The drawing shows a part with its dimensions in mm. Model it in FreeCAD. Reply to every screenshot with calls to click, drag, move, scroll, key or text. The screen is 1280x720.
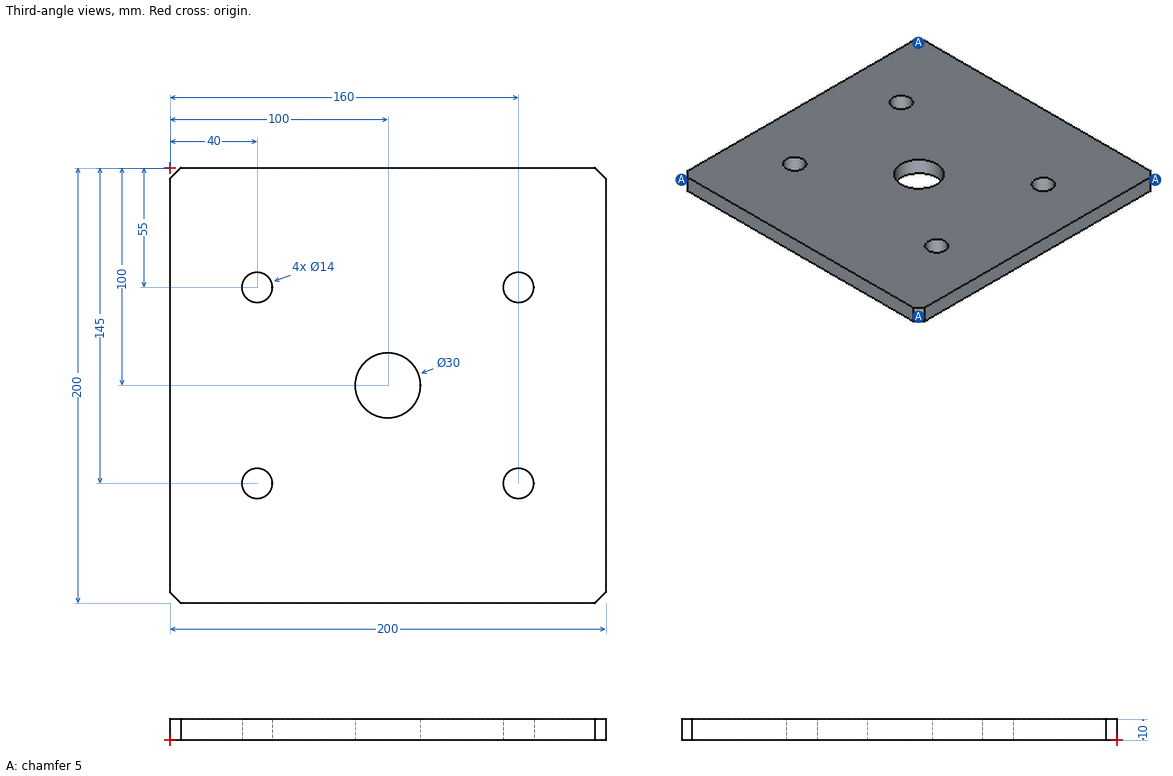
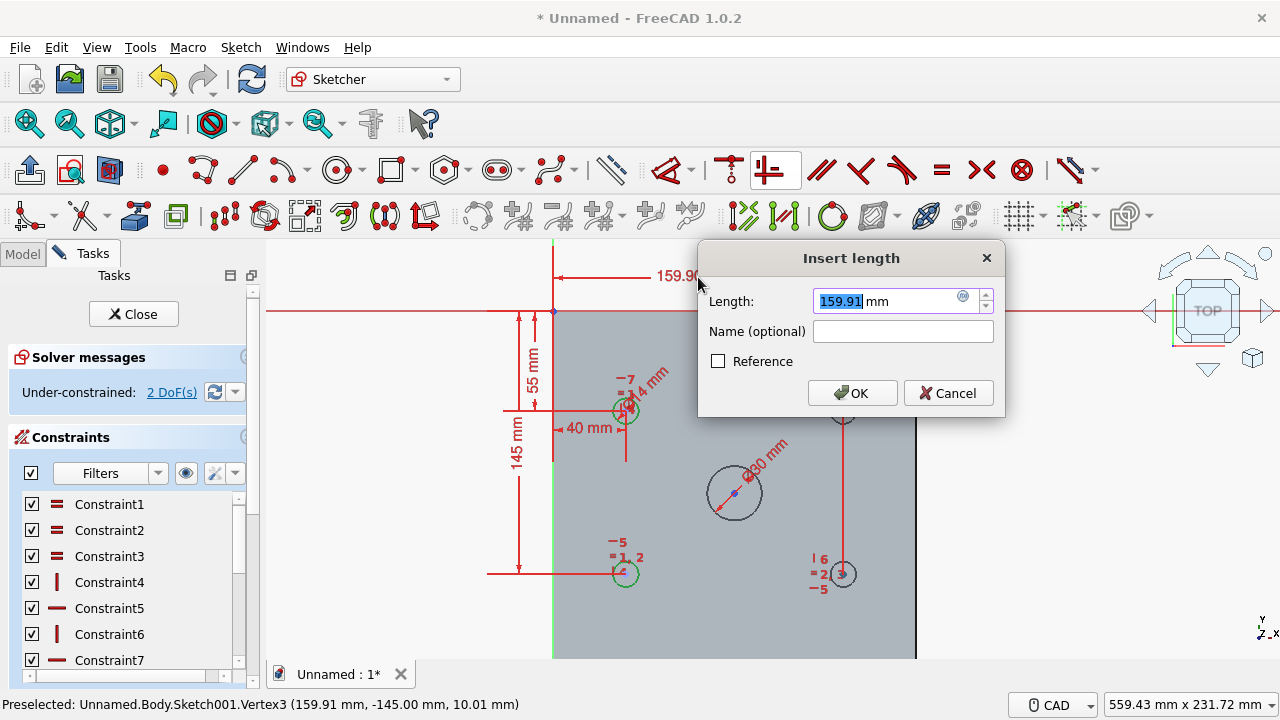
text(160)
key(Return)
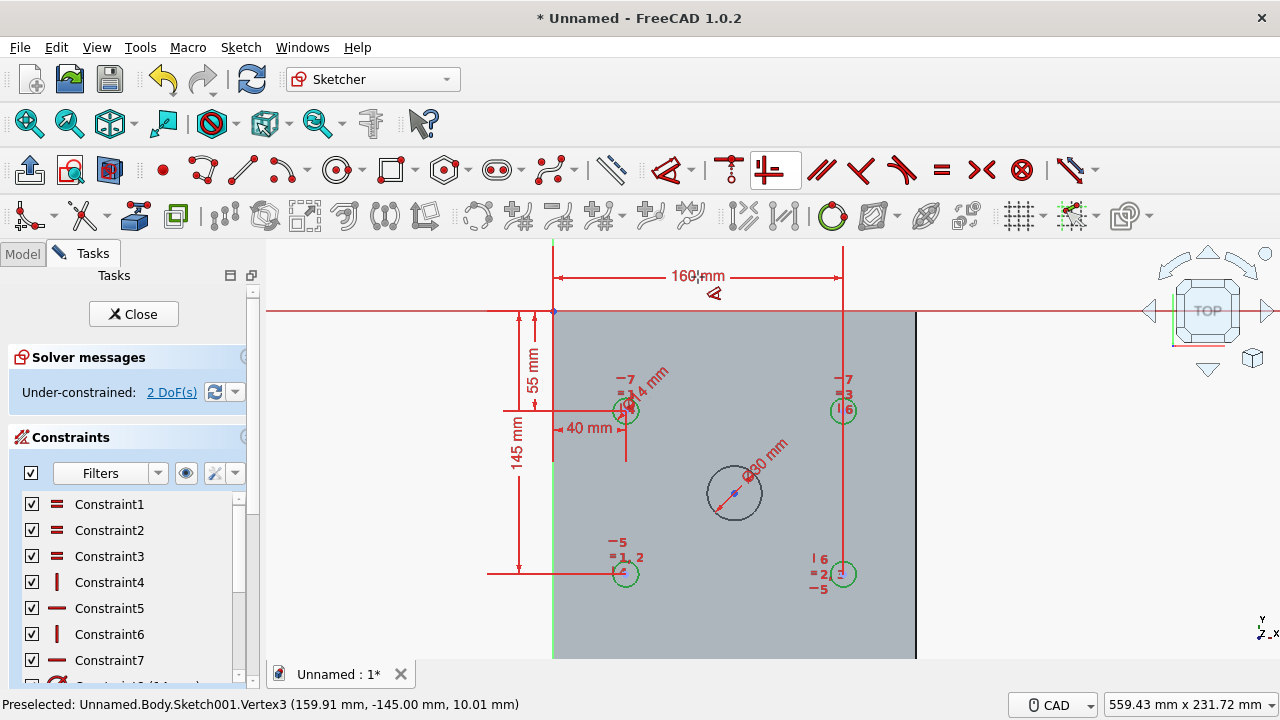
click(735, 493)
click(602, 277)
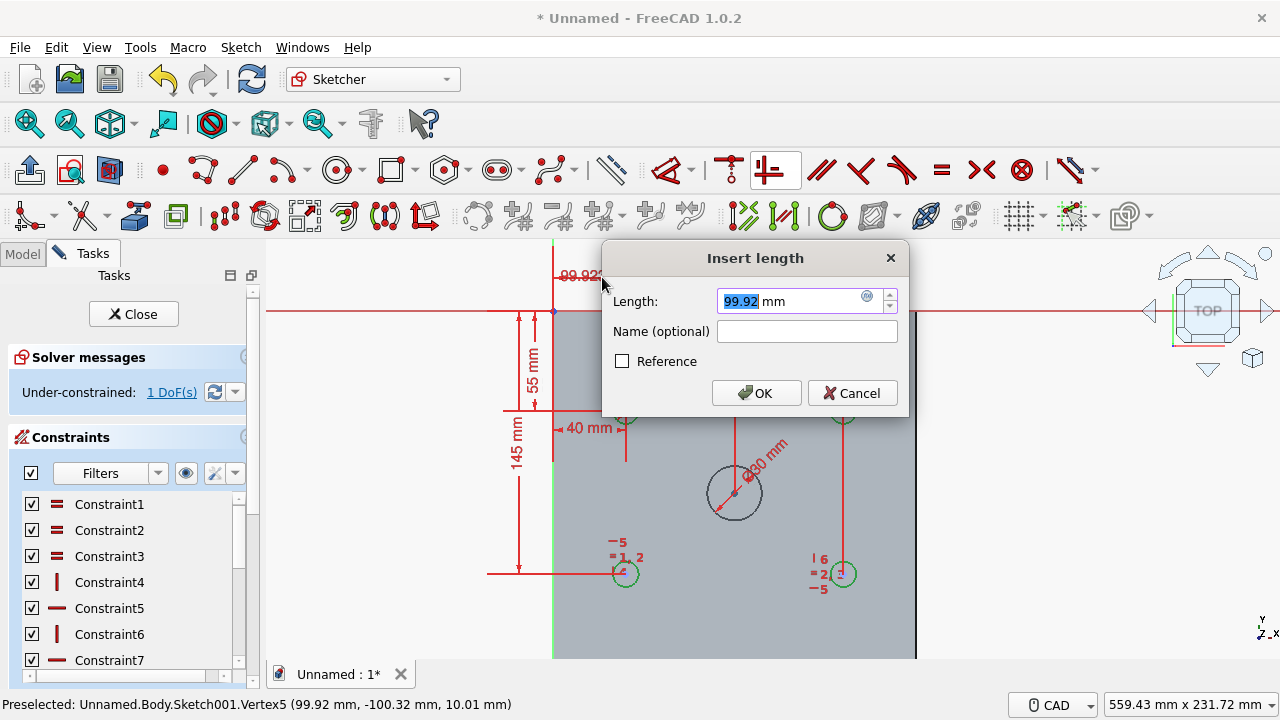
text(100)
key(Return)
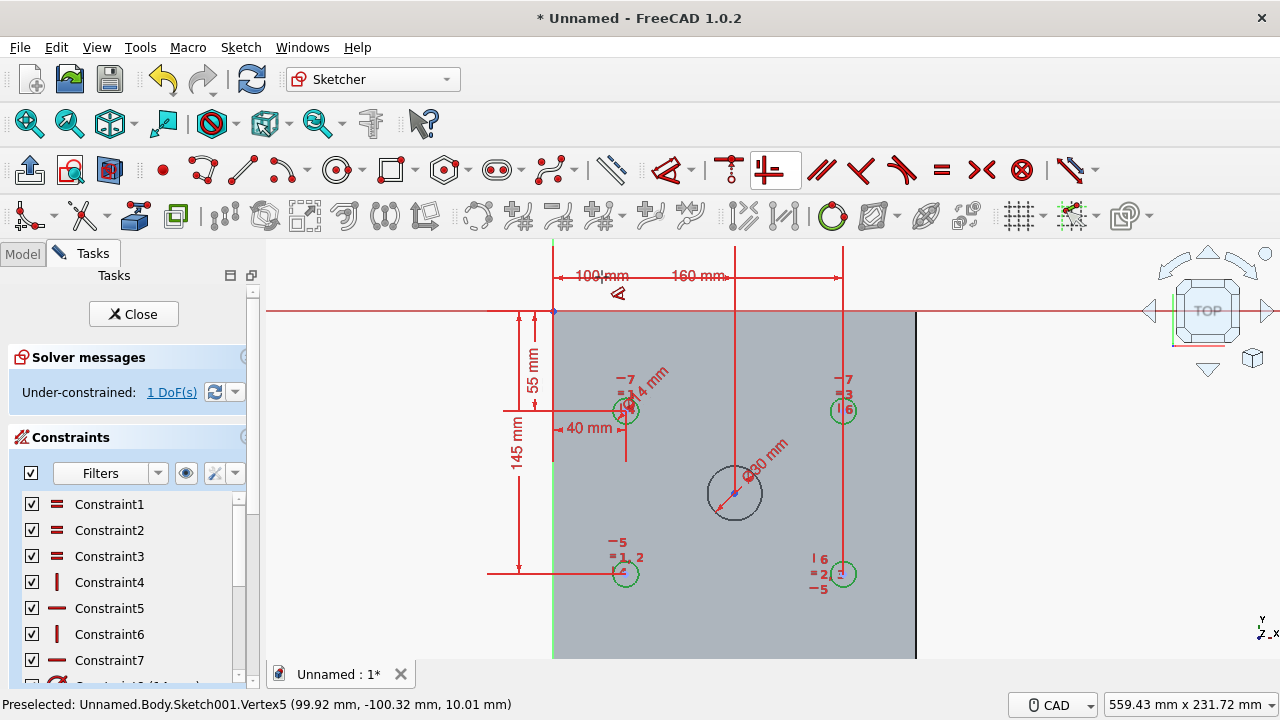
click(735, 493)
click(519, 402)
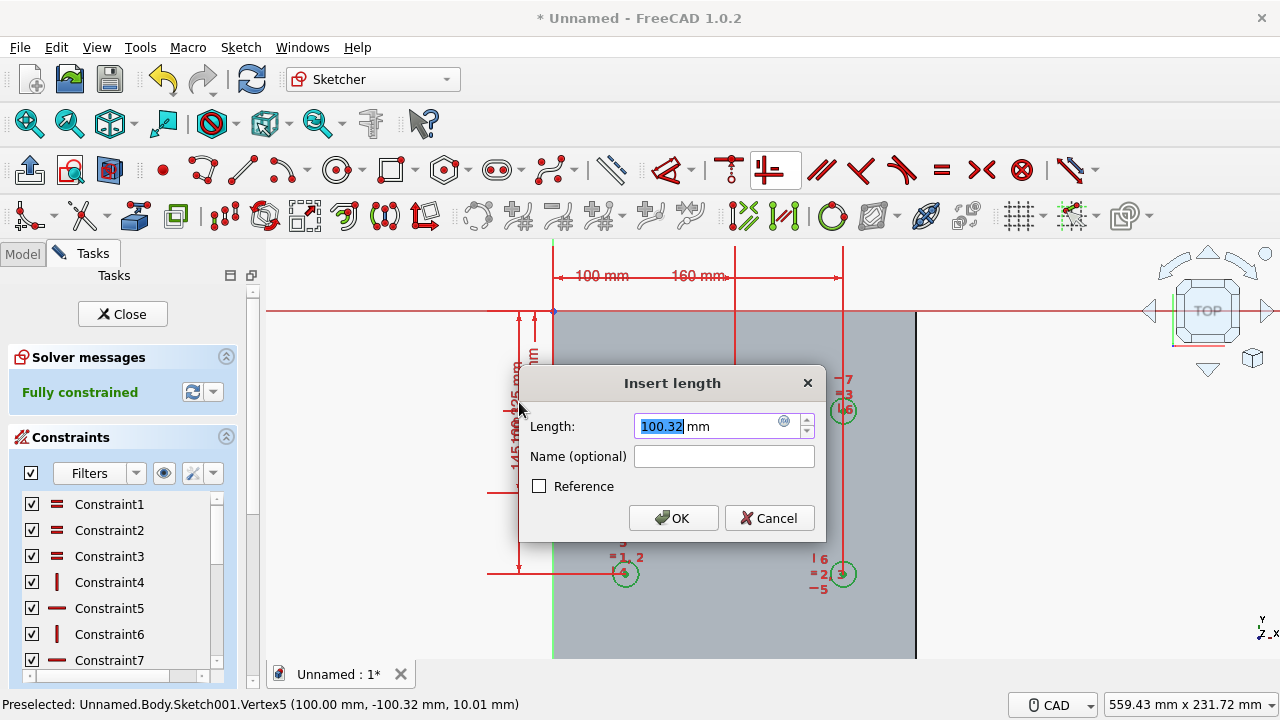
text(100)
key(Return)
key(Escape)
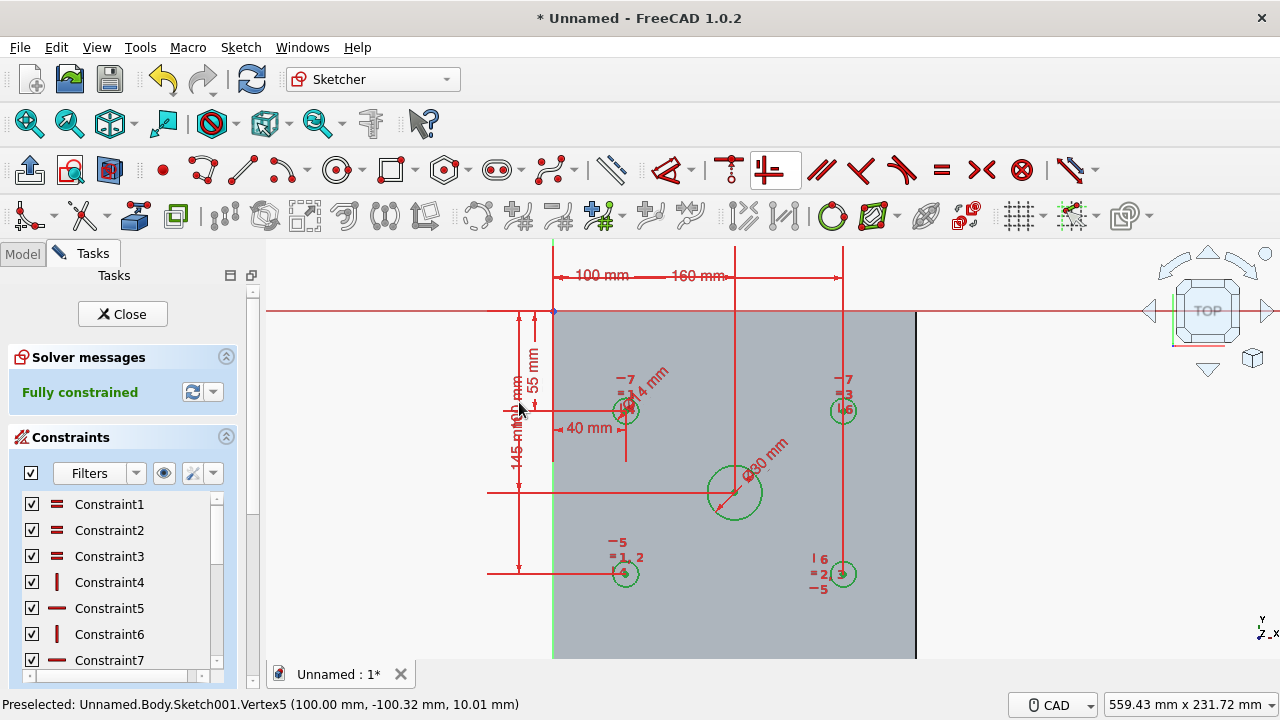
click(123, 314)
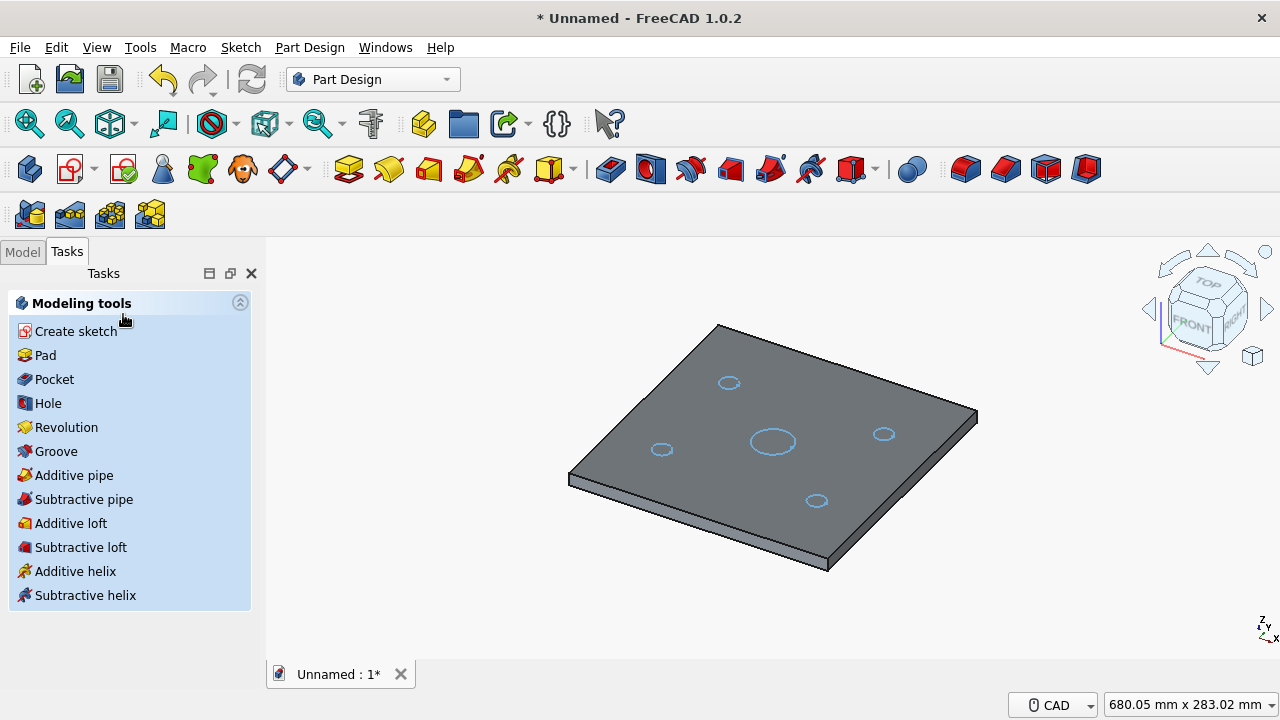
click(612, 170)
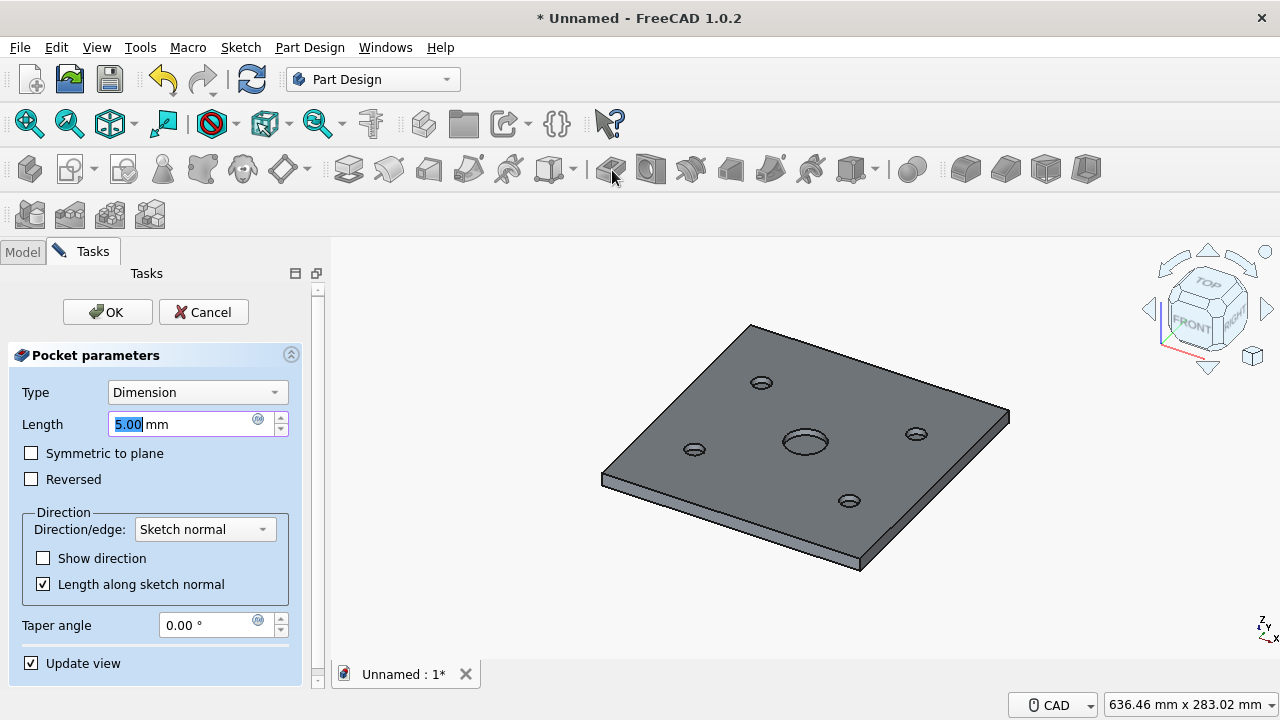
click(198, 392)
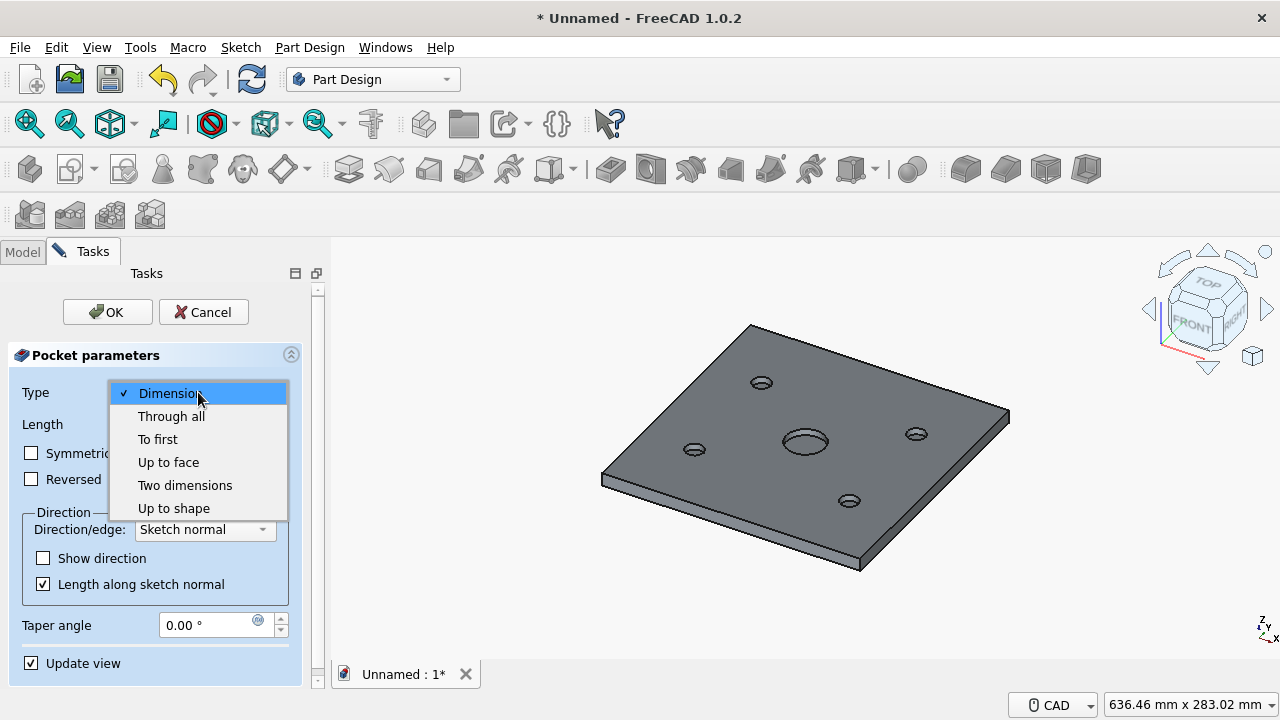
click(198, 416)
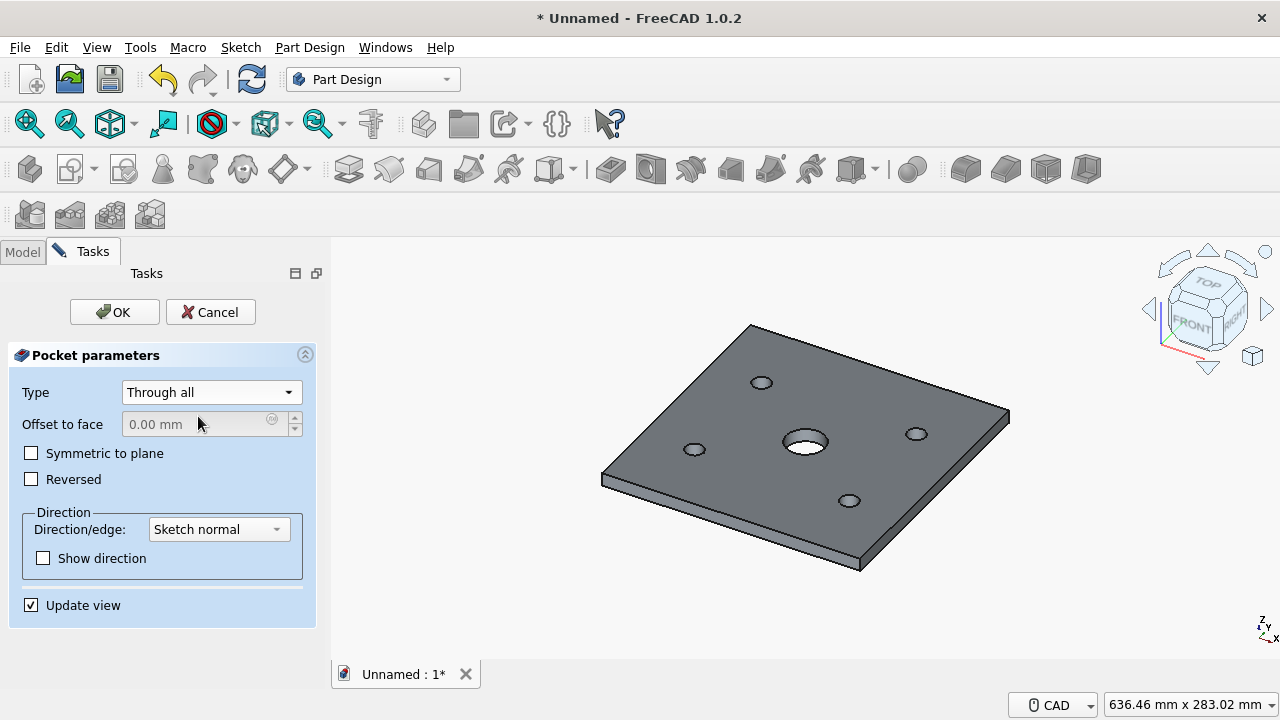
click(115, 312)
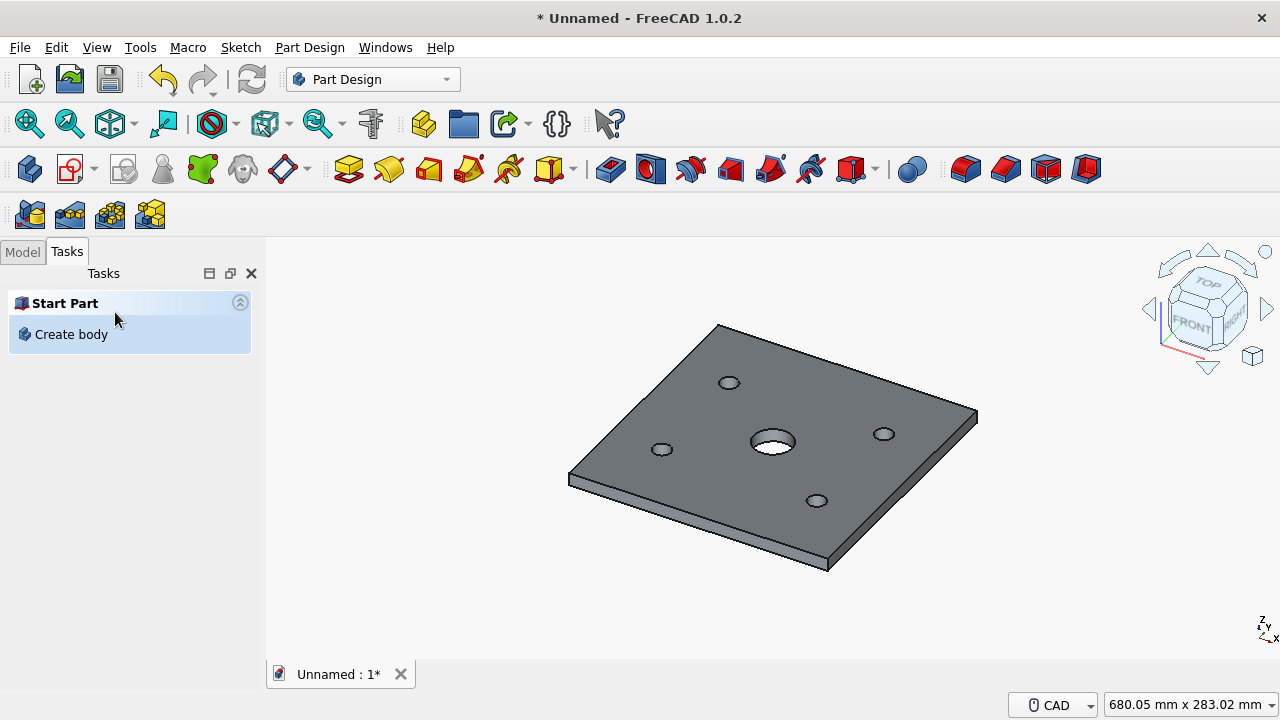
click(828, 564)